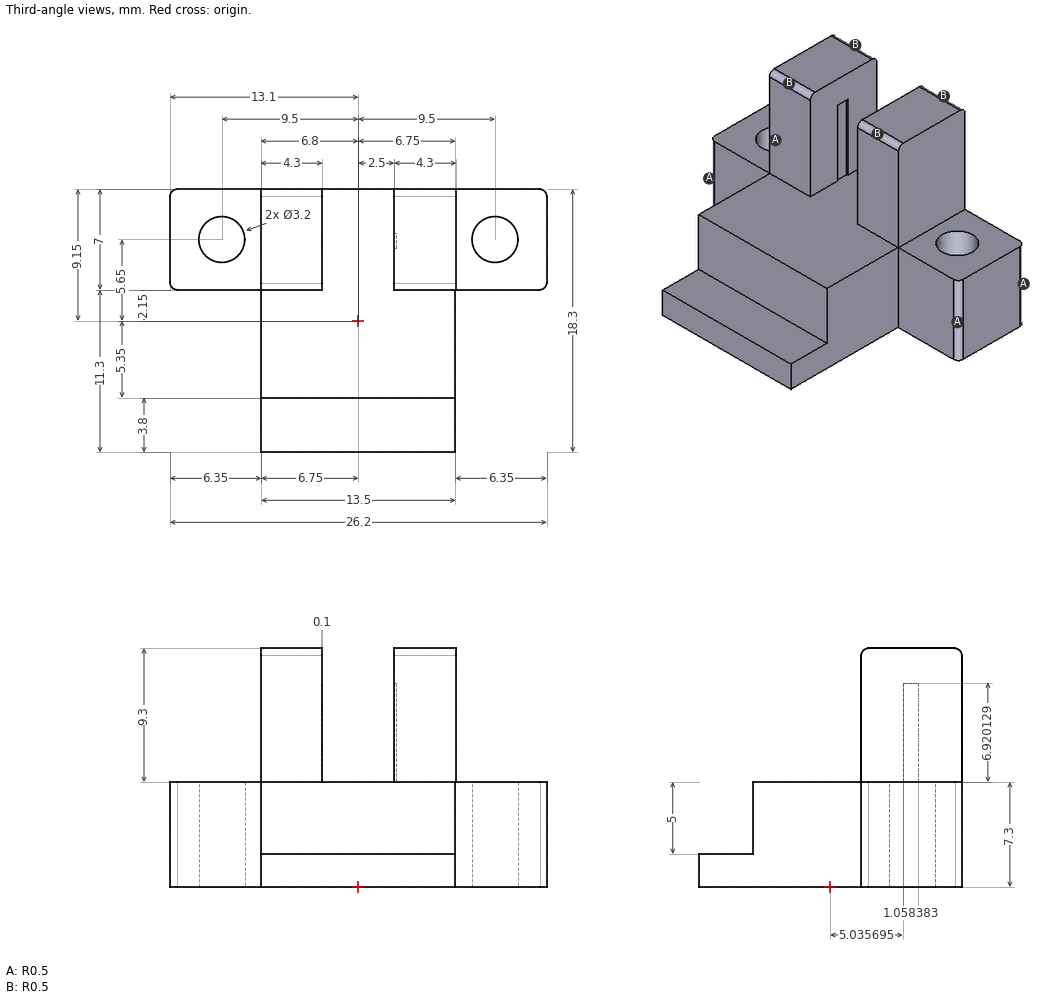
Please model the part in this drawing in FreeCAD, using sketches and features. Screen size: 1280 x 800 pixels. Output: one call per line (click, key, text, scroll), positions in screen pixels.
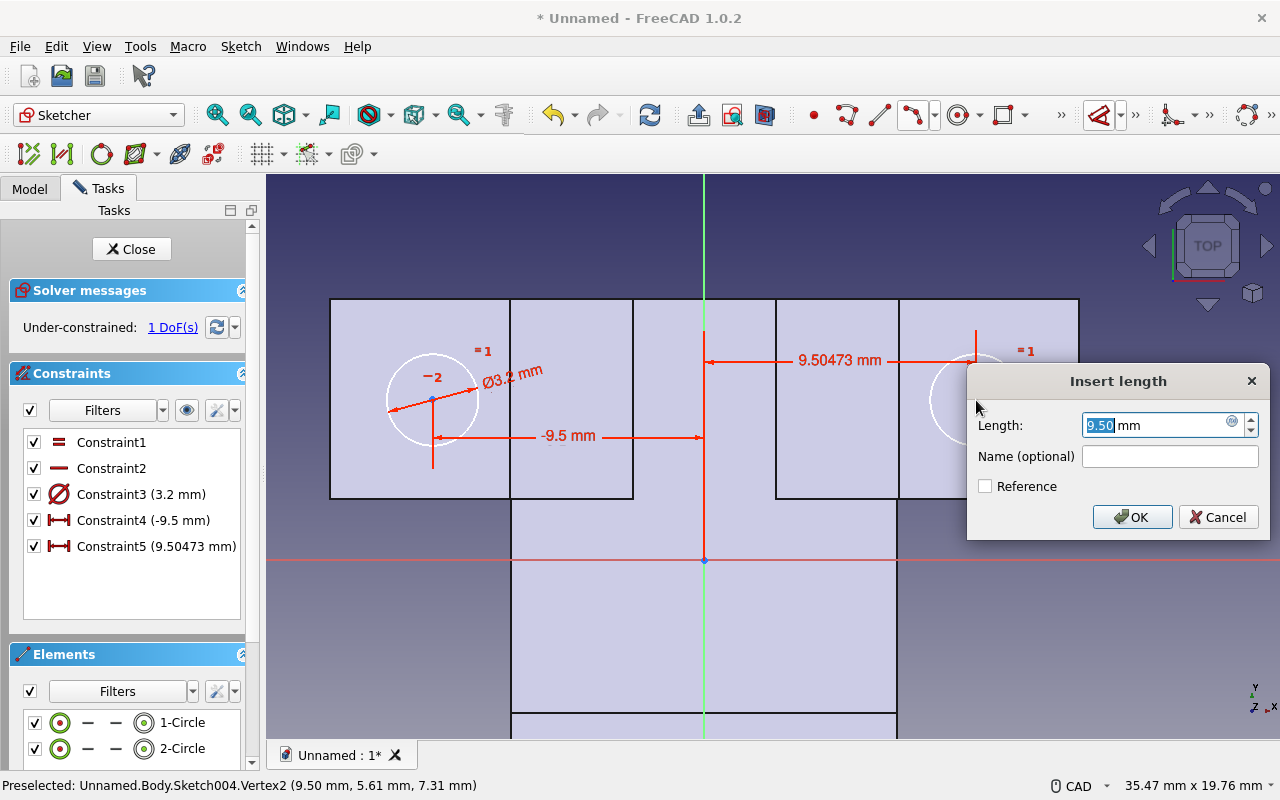
text(9.5)
key(Return)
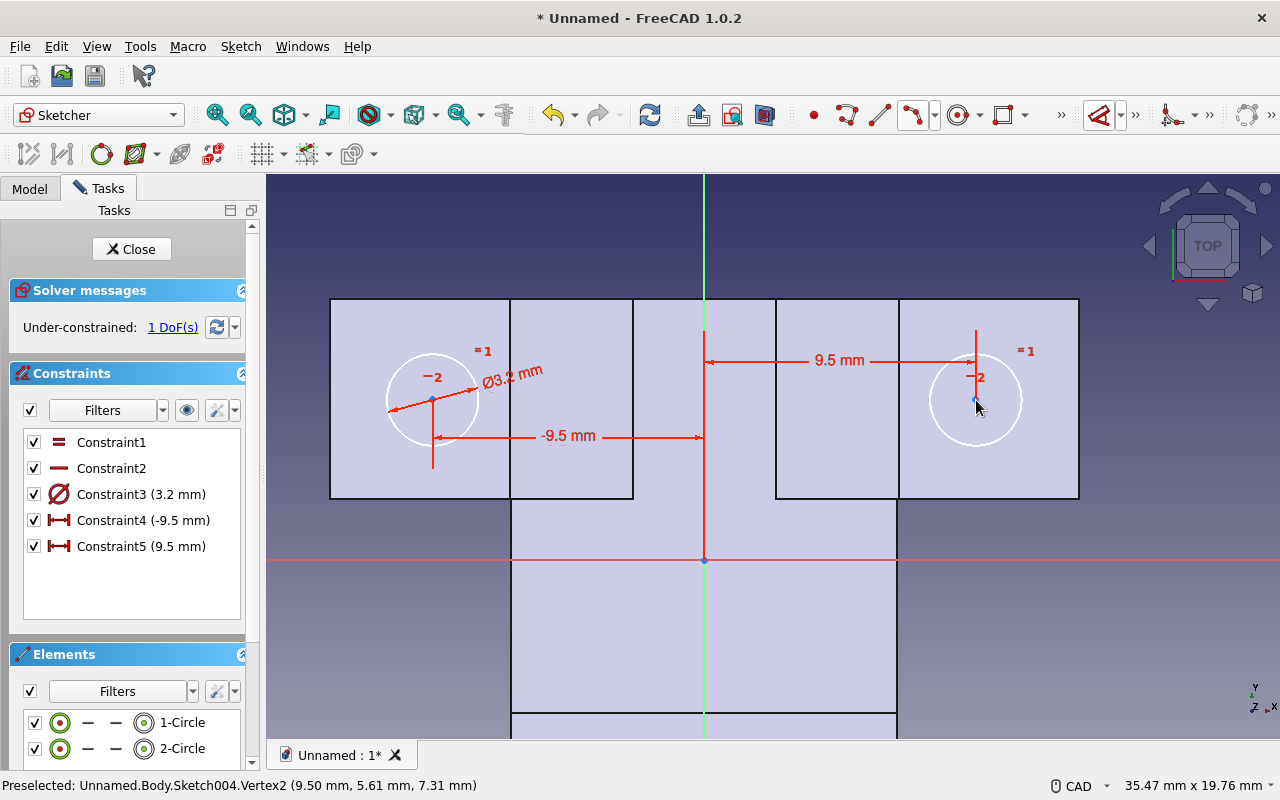
click(433, 400)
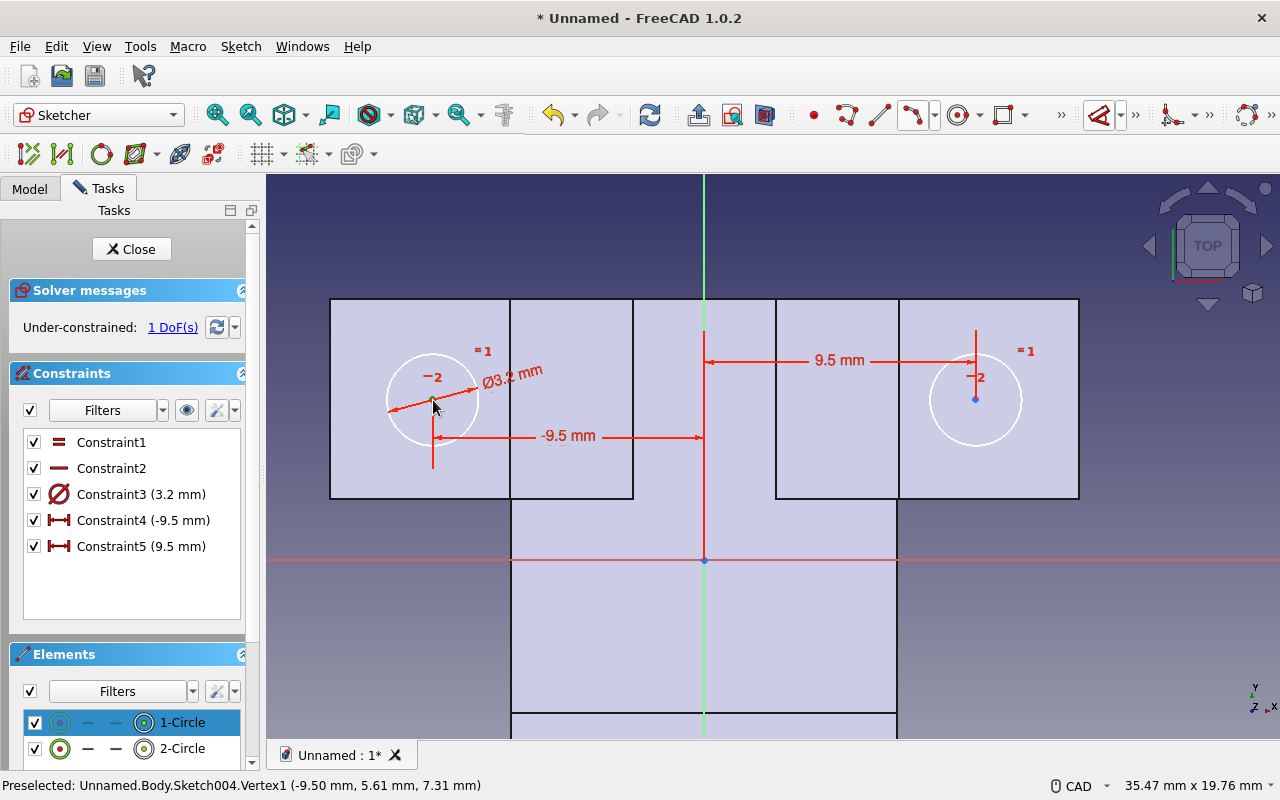
key(i)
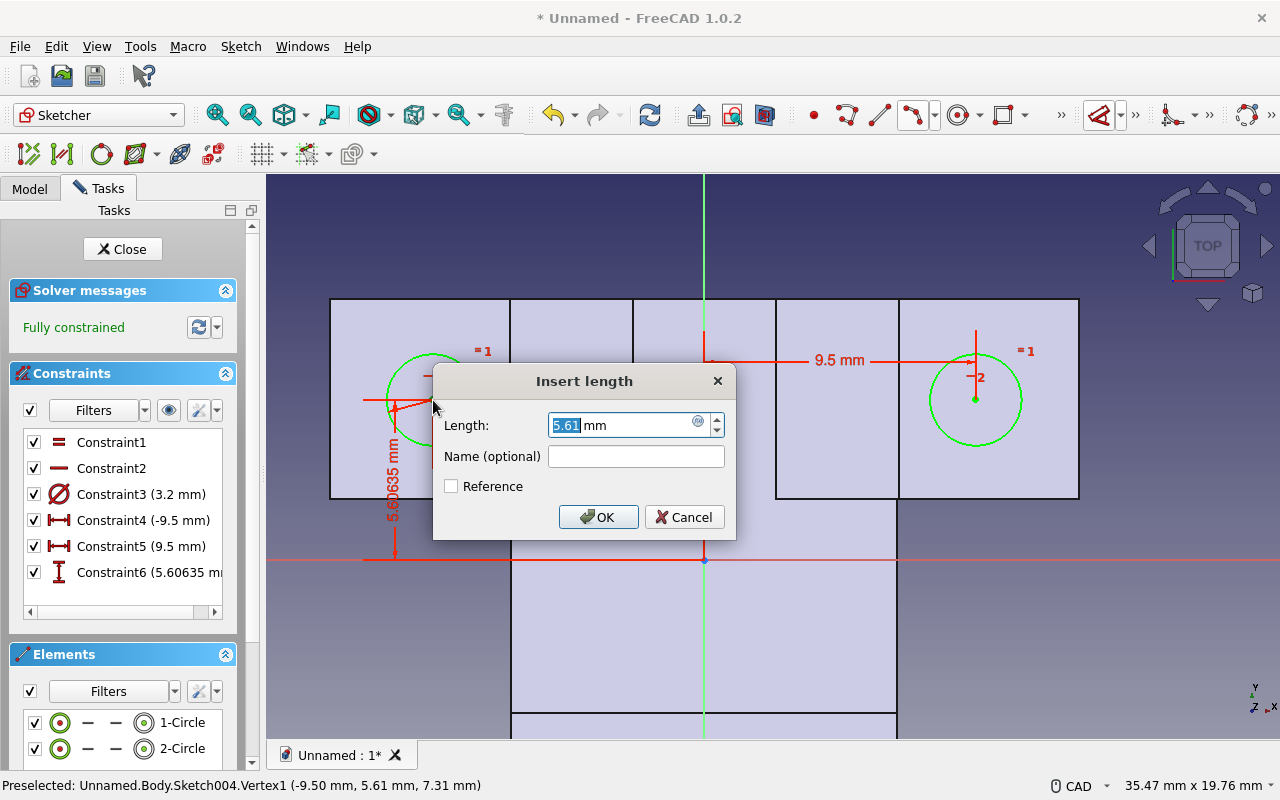
text(5.65)
key(Return)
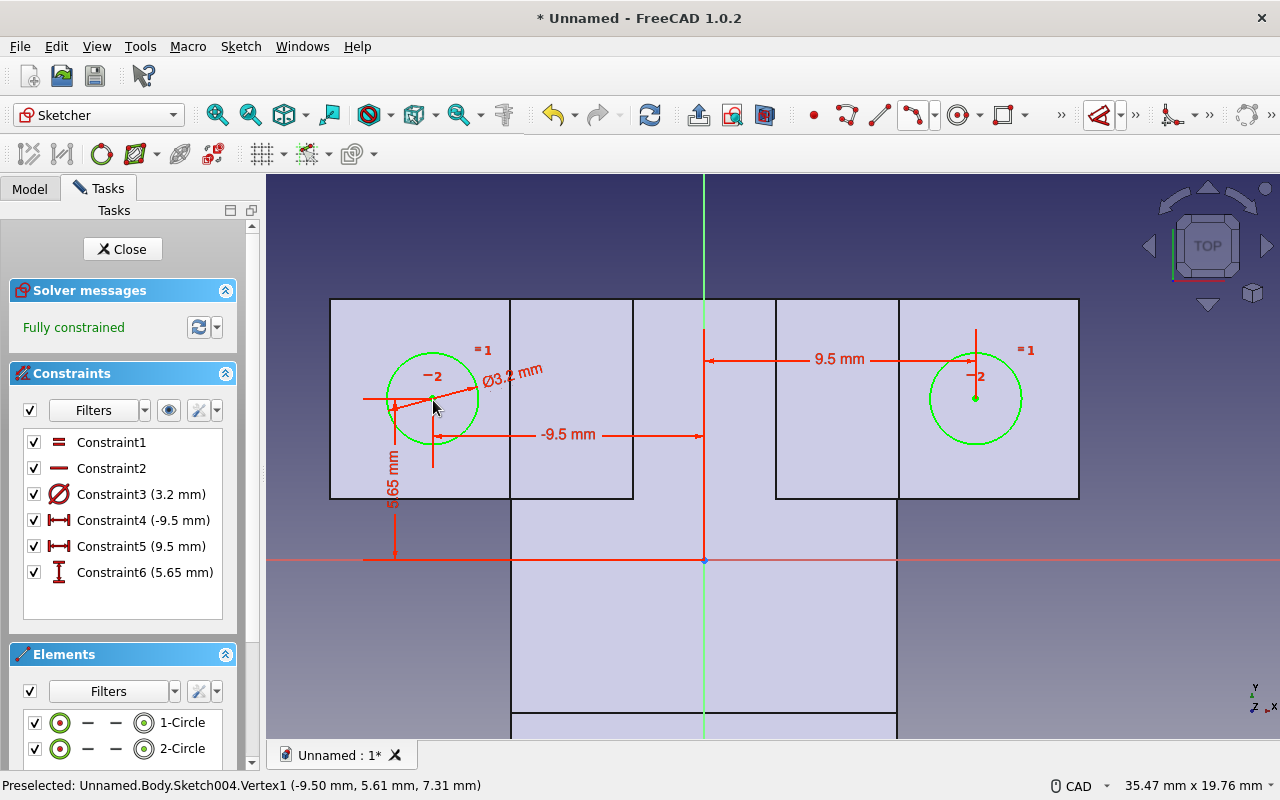
click(123, 249)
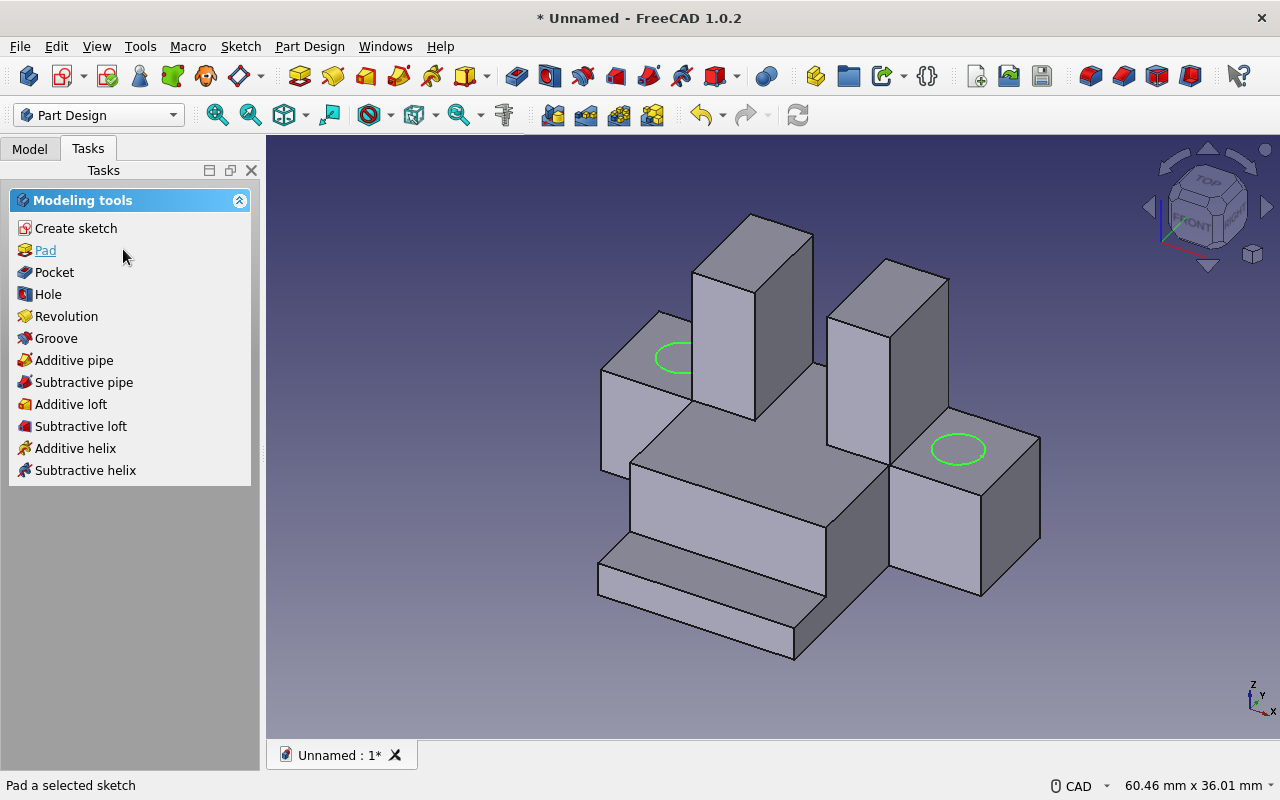
click(517, 76)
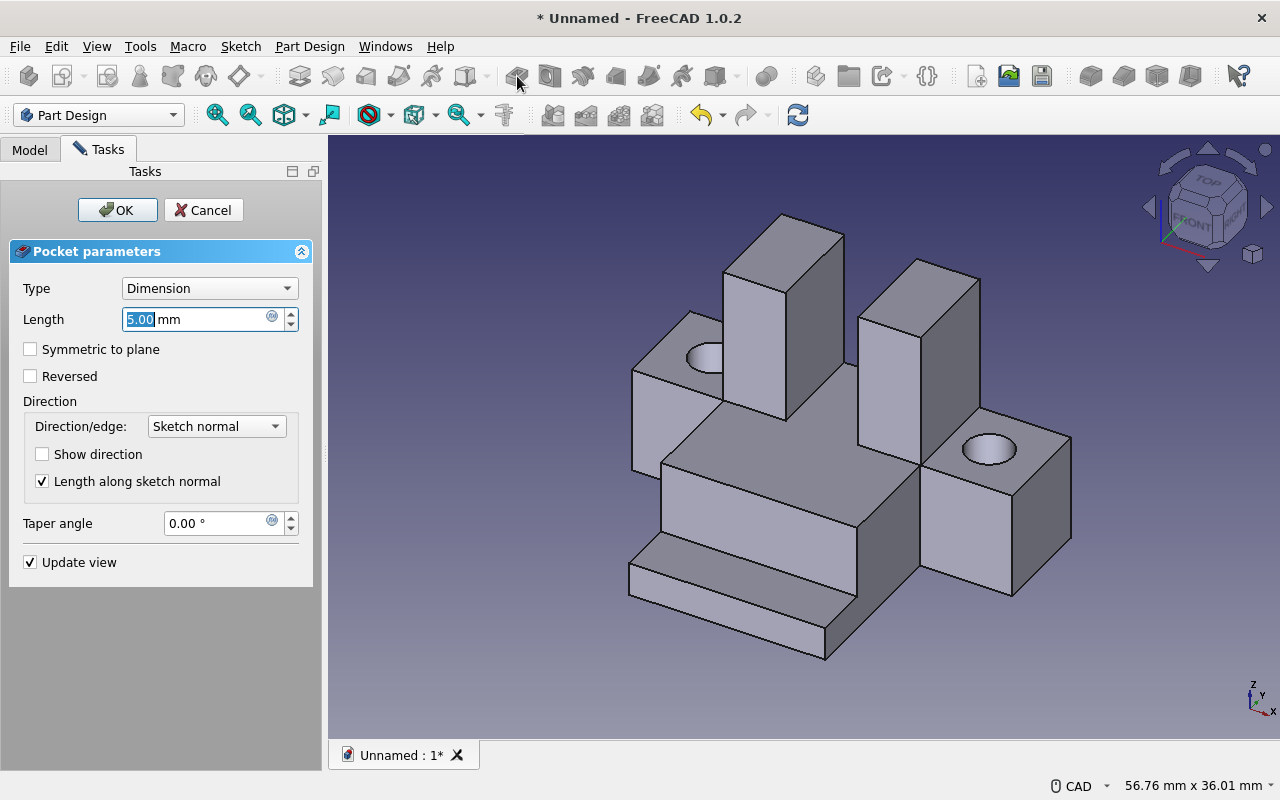
click(210, 288)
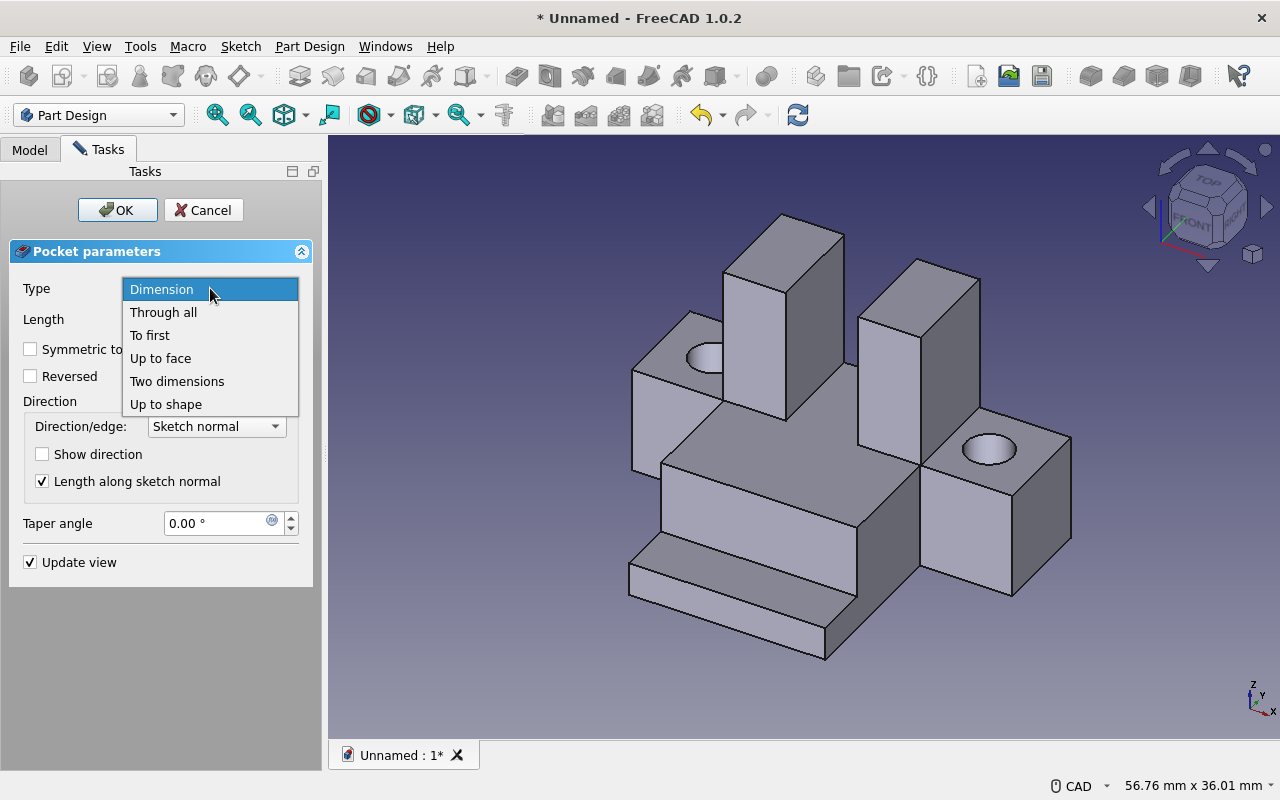
click(208, 312)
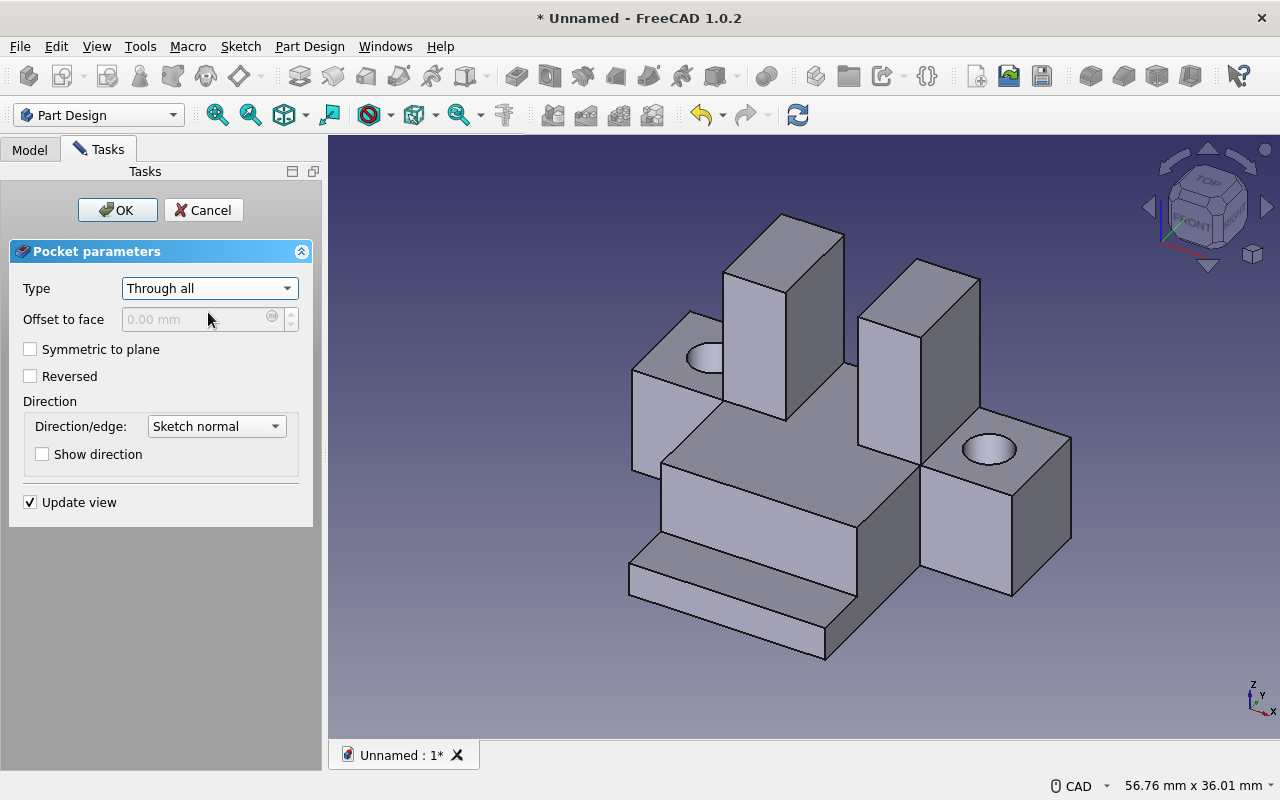
click(118, 210)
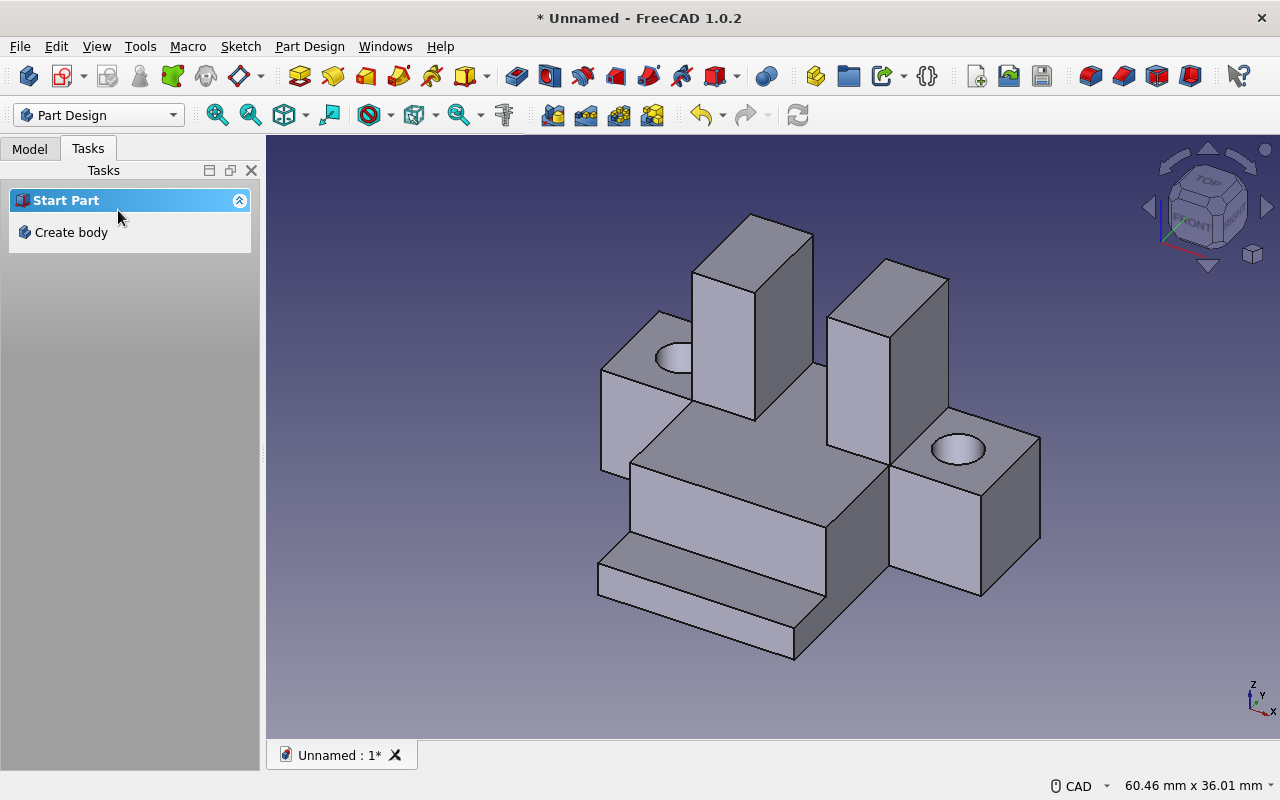
click(30, 148)